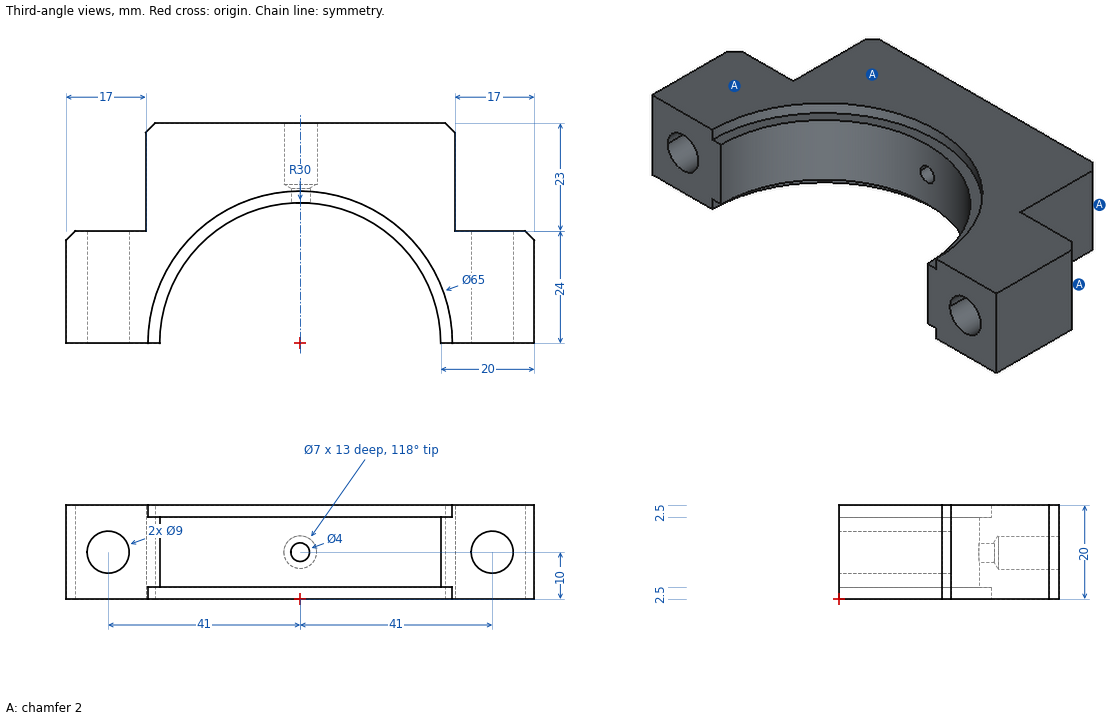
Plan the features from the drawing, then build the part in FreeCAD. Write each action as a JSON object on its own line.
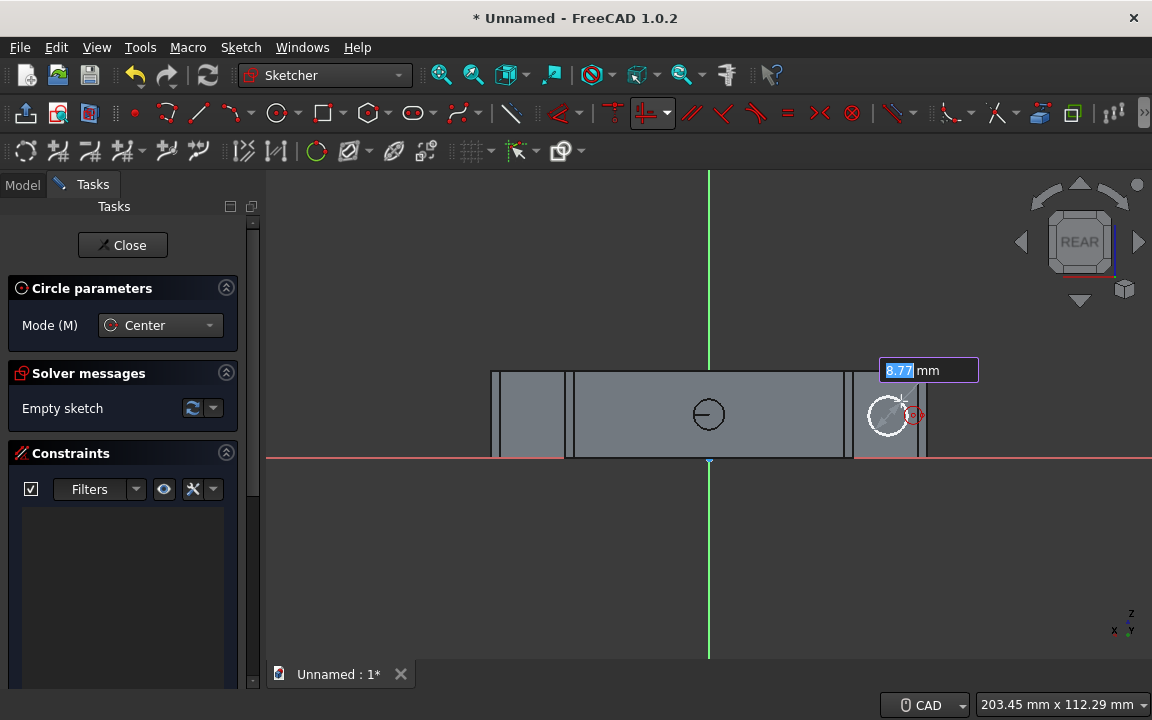
{"action": "type", "text": "9"}
{"action": "key", "text": "Return"}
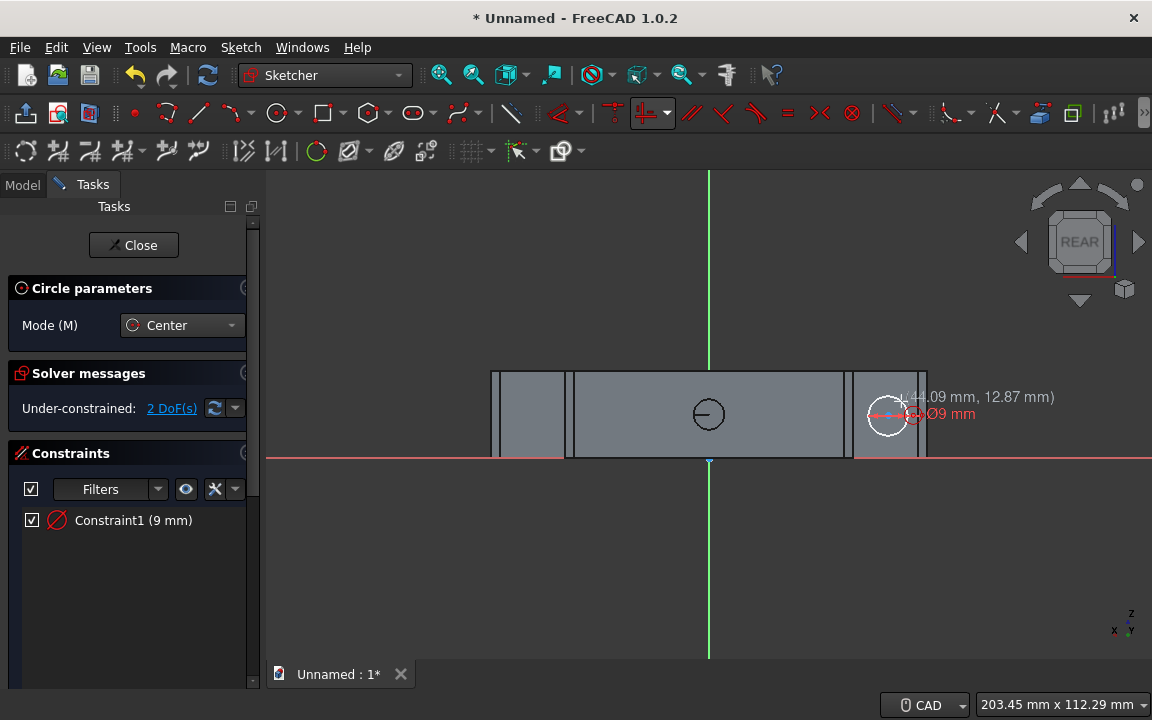
{"action": "left_click", "coordinate": [530, 415]}
{"action": "mouse_move", "coordinate": [544, 401]}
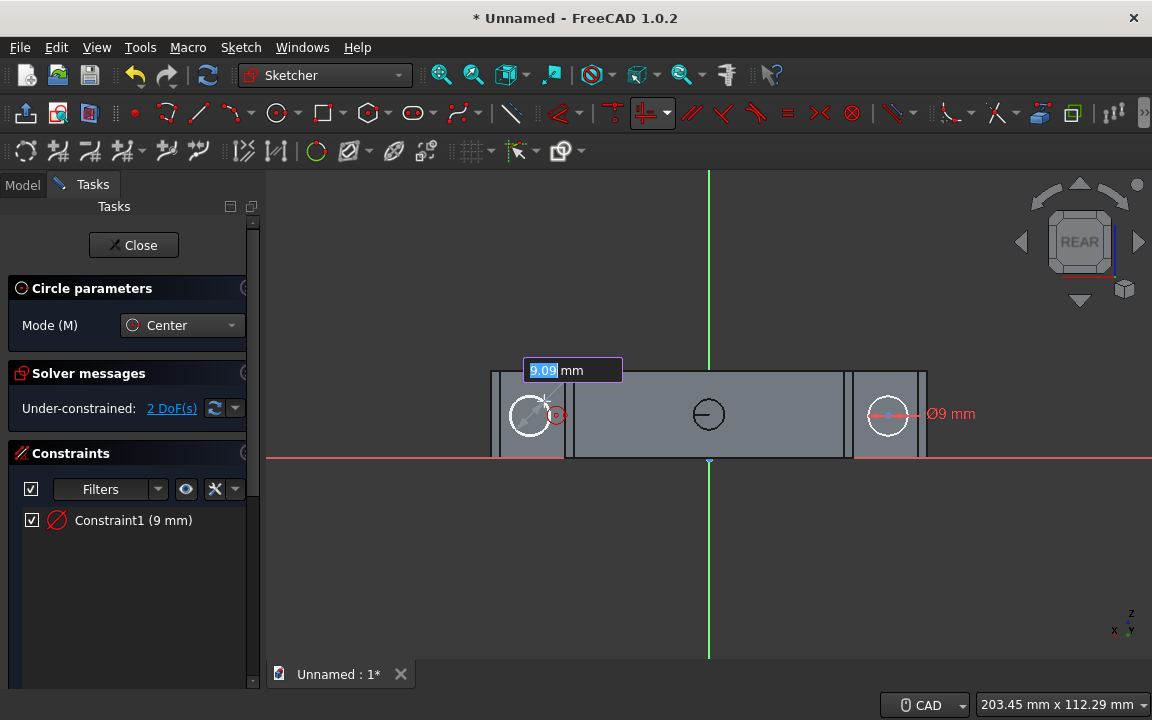
{"action": "type", "text": "9"}
{"action": "key", "text": "Return"}
{"action": "key", "text": "Escape"}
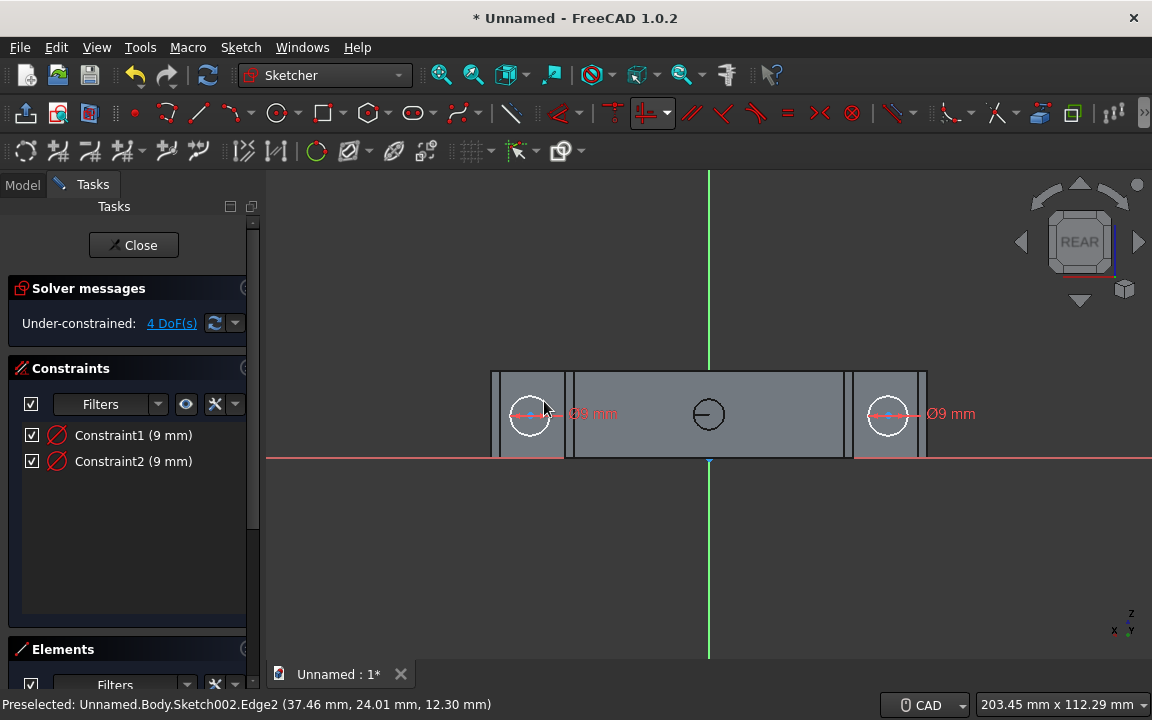
{"action": "left_click", "coordinate": [888, 416]}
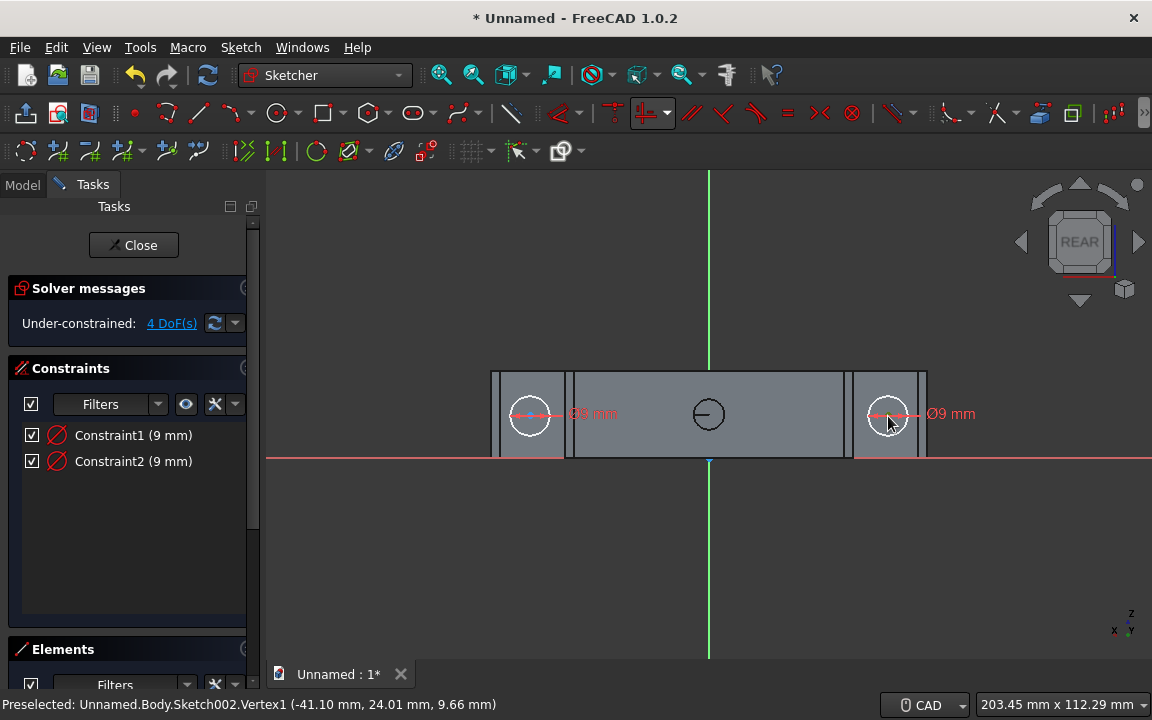
{"action": "left_click", "coordinate": [530, 416]}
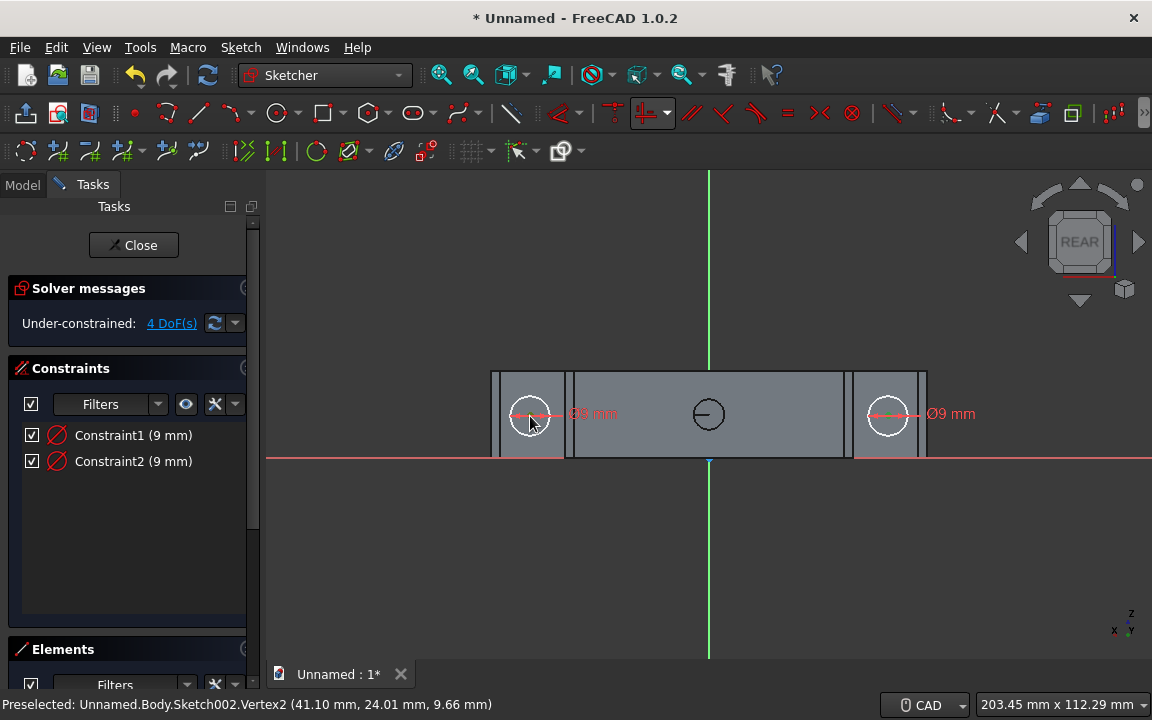
{"action": "left_click", "coordinate": [670, 114]}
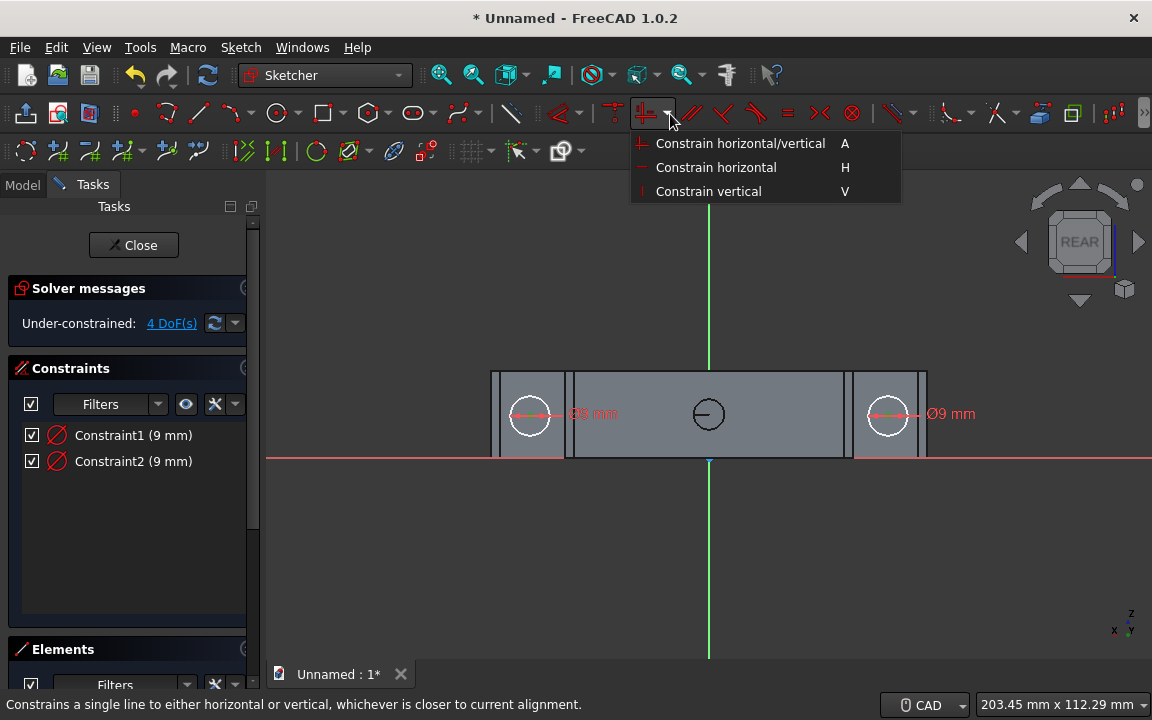
{"action": "left_click", "coordinate": [766, 167]}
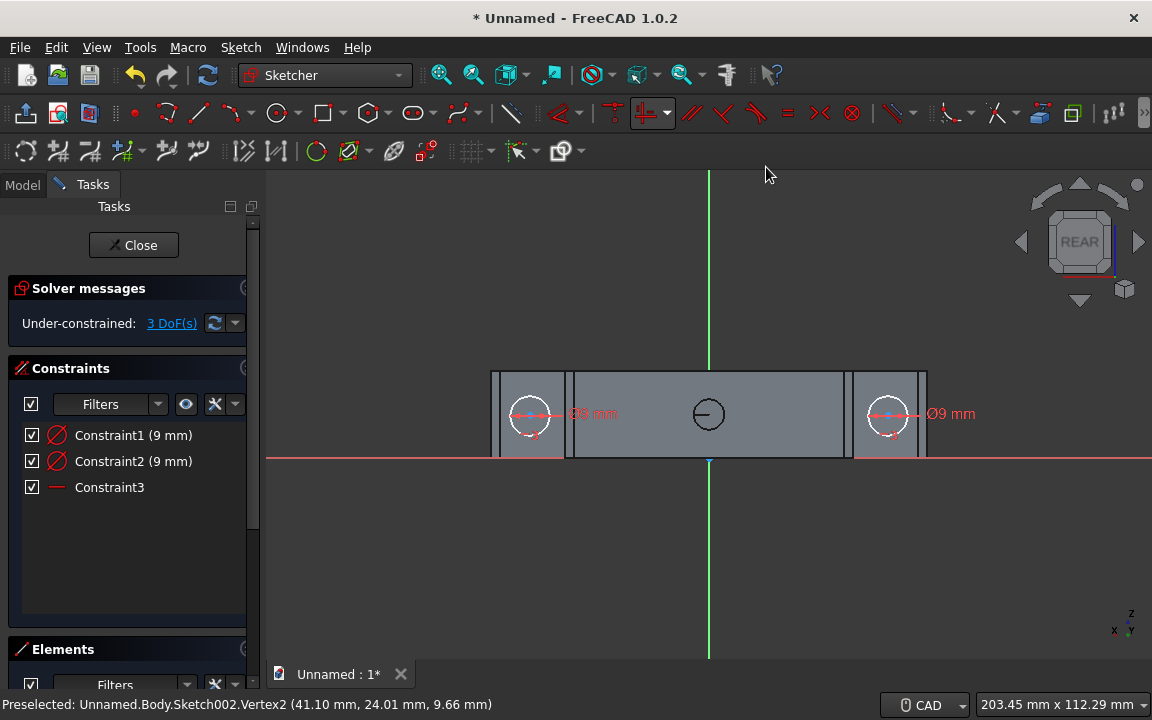
{"action": "left_click", "coordinate": [558, 114]}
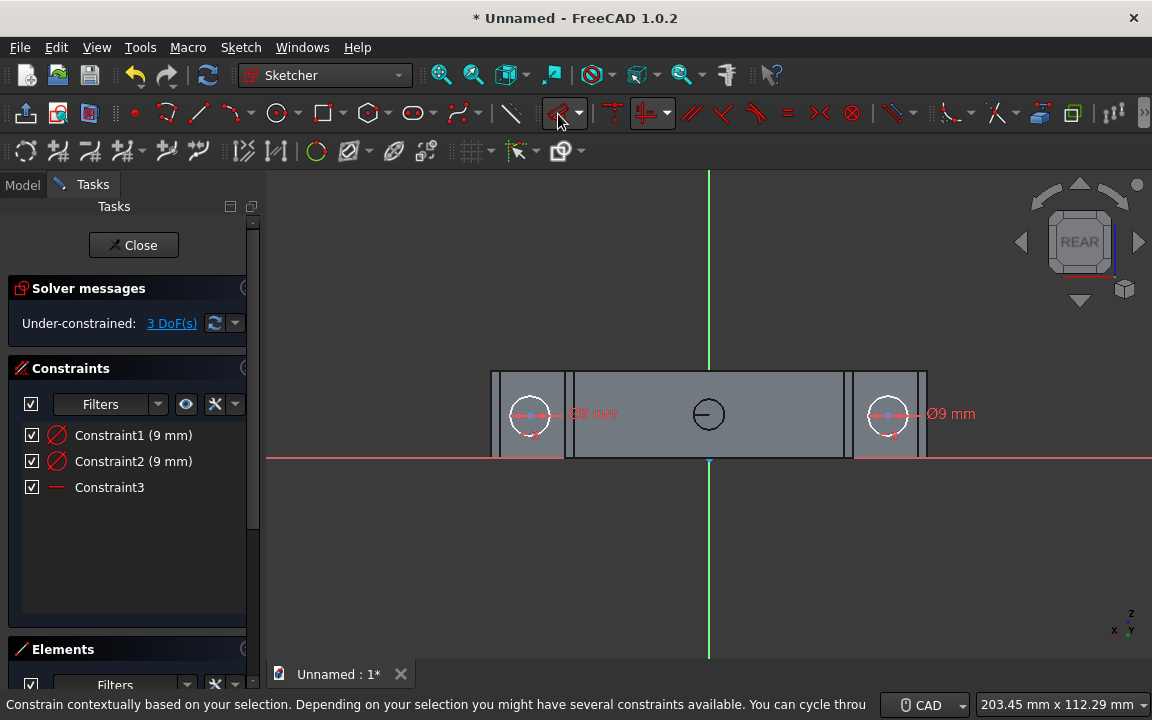
{"action": "left_click", "coordinate": [888, 416]}
{"action": "left_click", "coordinate": [799, 492]}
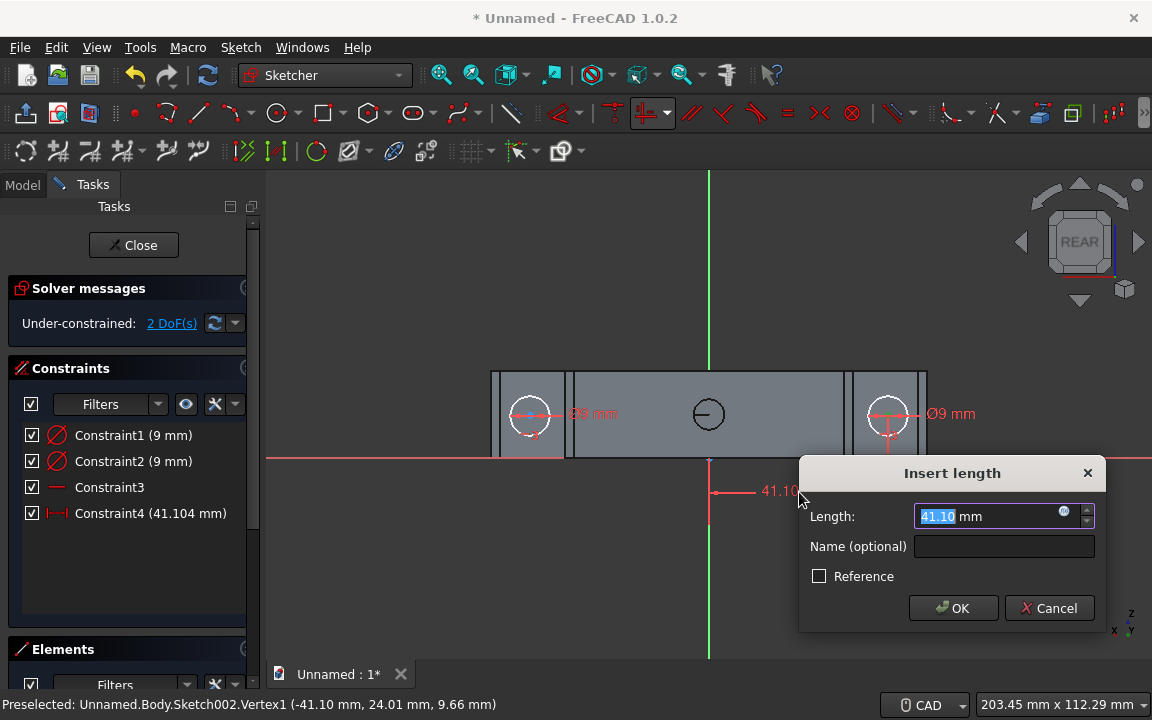
{"action": "type", "text": "41"}
{"action": "key", "text": "Return"}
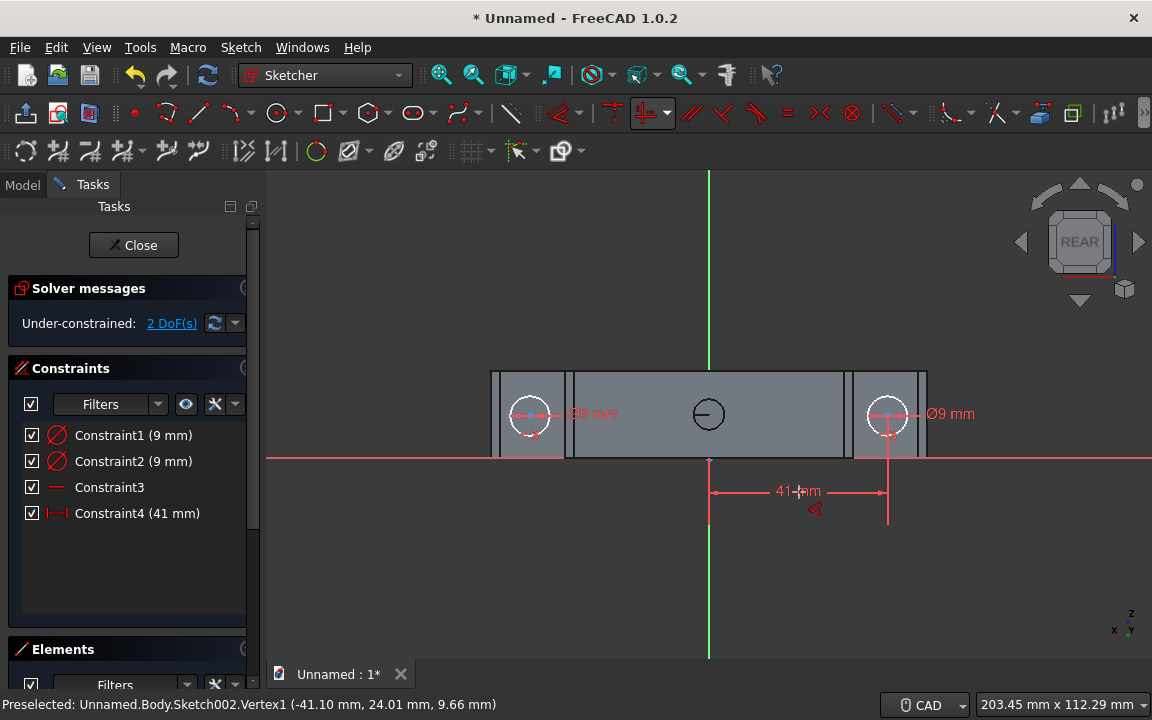
{"action": "left_click", "coordinate": [888, 416]}
{"action": "left_click", "coordinate": [922, 437]}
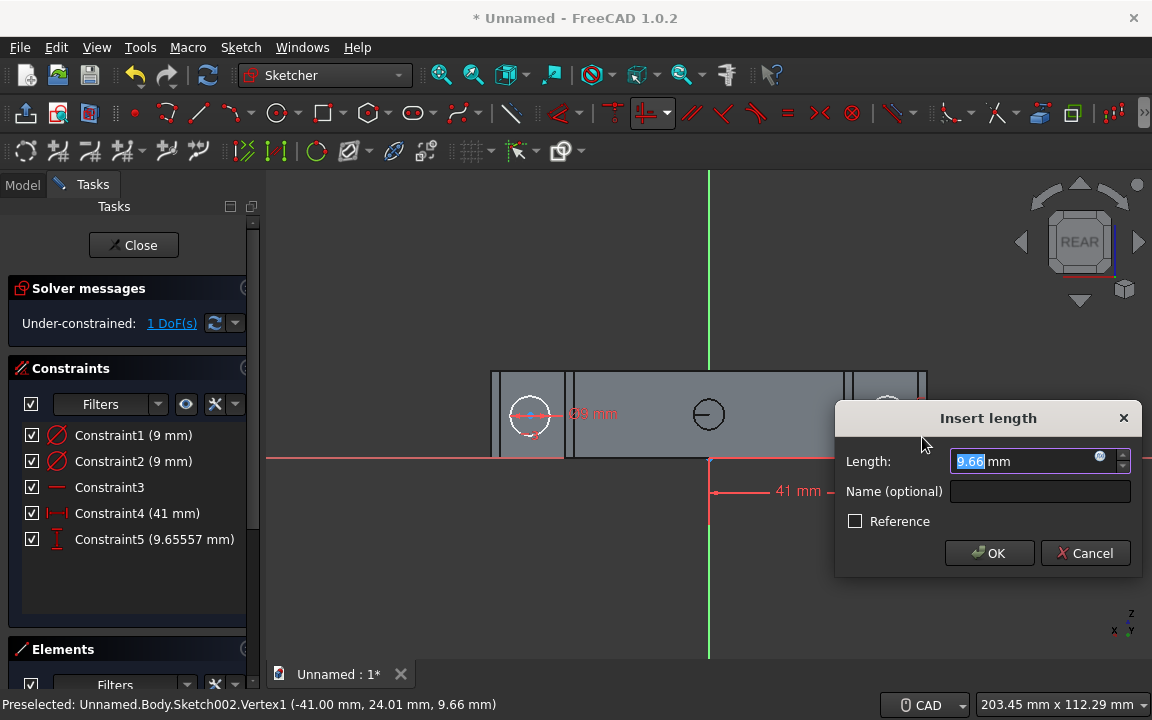
{"action": "type", "text": "10"}
{"action": "key", "text": "Return"}